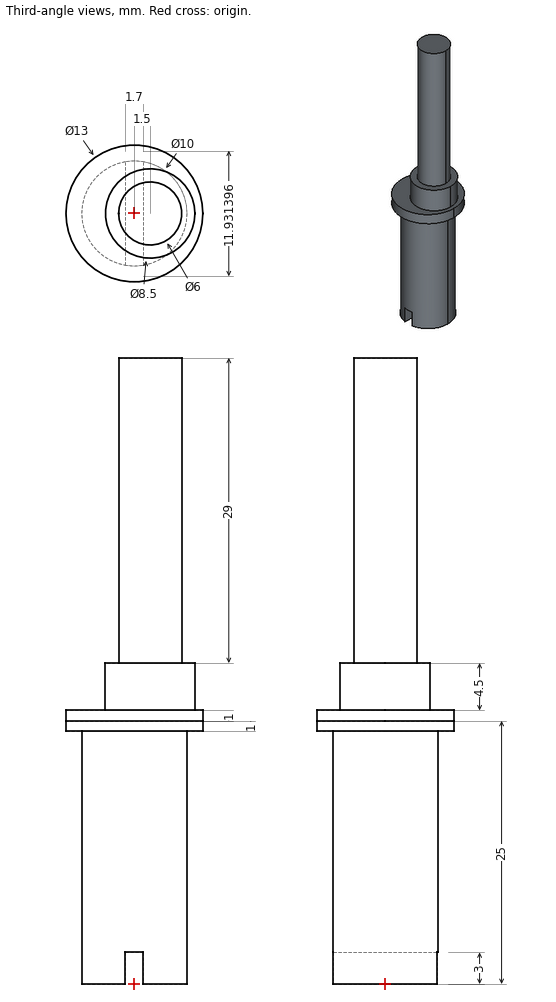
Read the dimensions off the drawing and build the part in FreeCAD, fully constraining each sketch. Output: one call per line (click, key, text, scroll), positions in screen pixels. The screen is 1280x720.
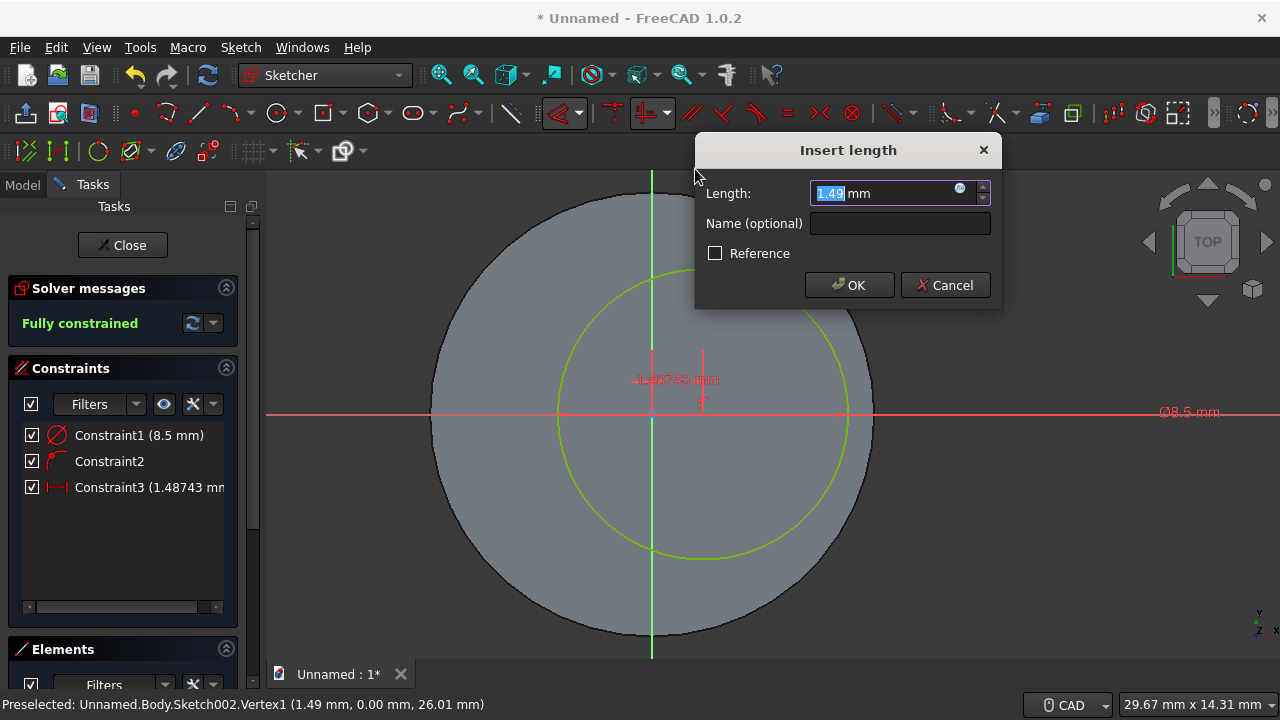
text(1.5)
key(Return)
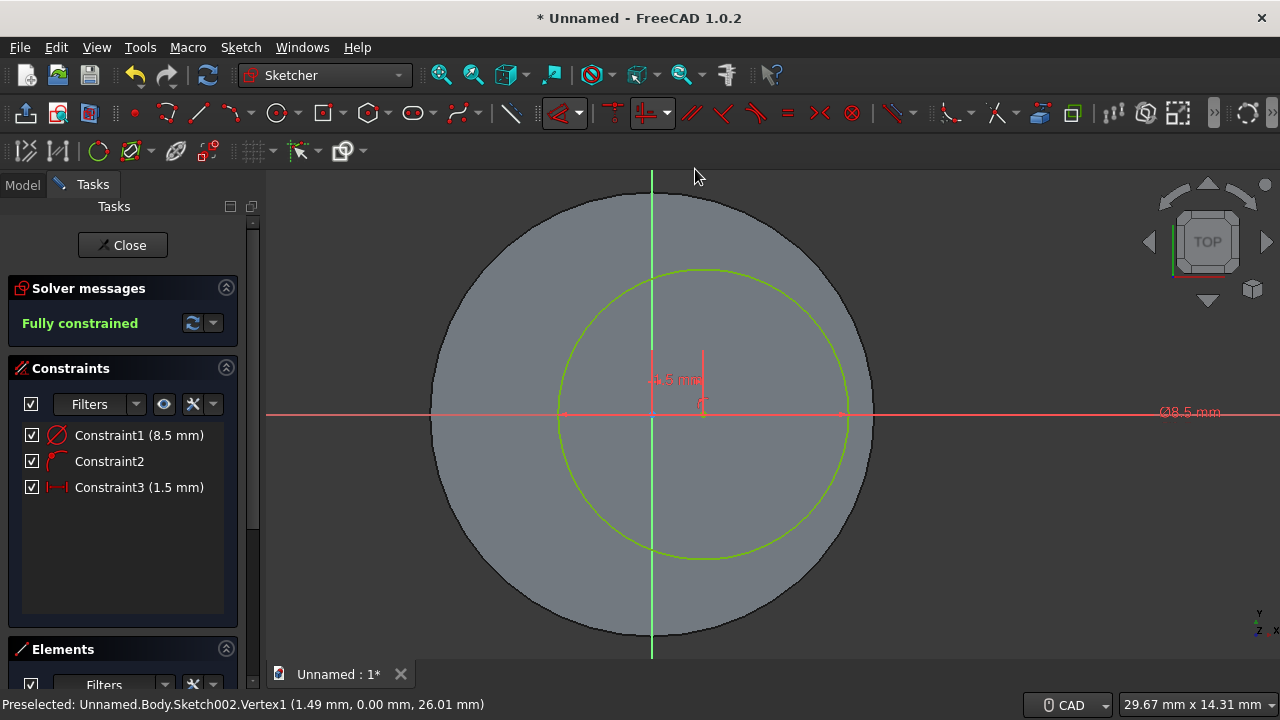
click(123, 245)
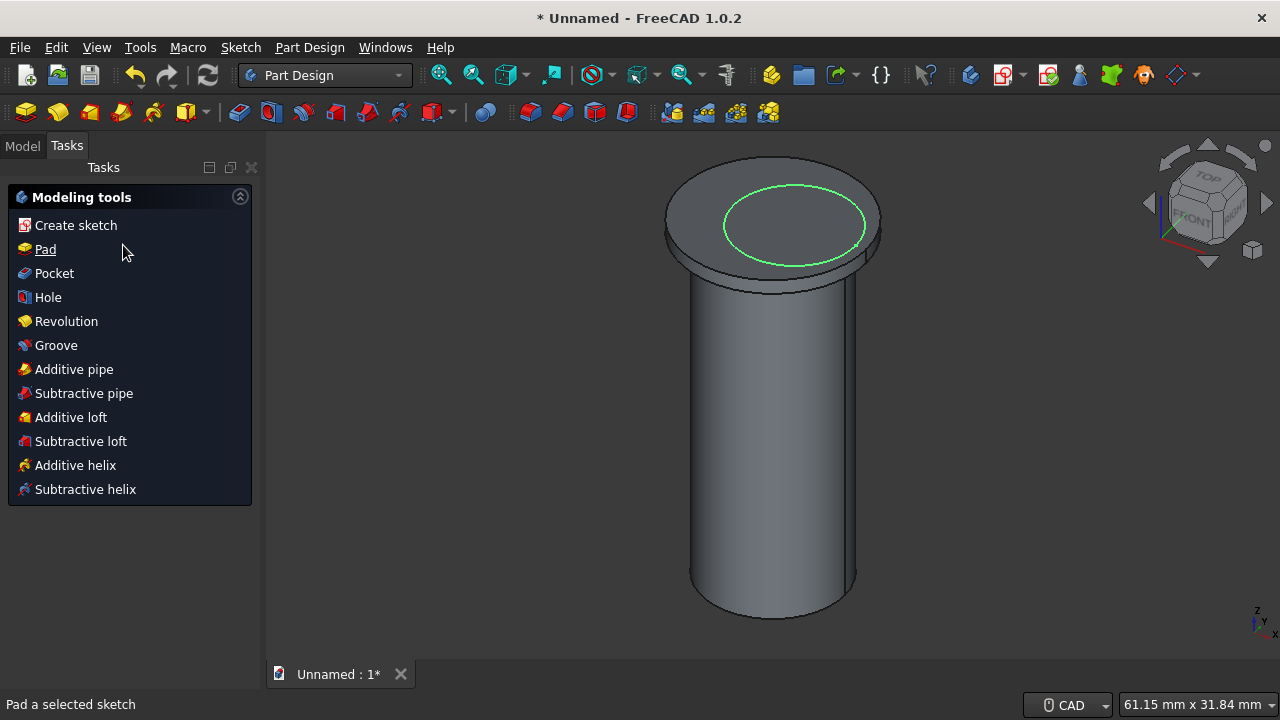
click(26, 112)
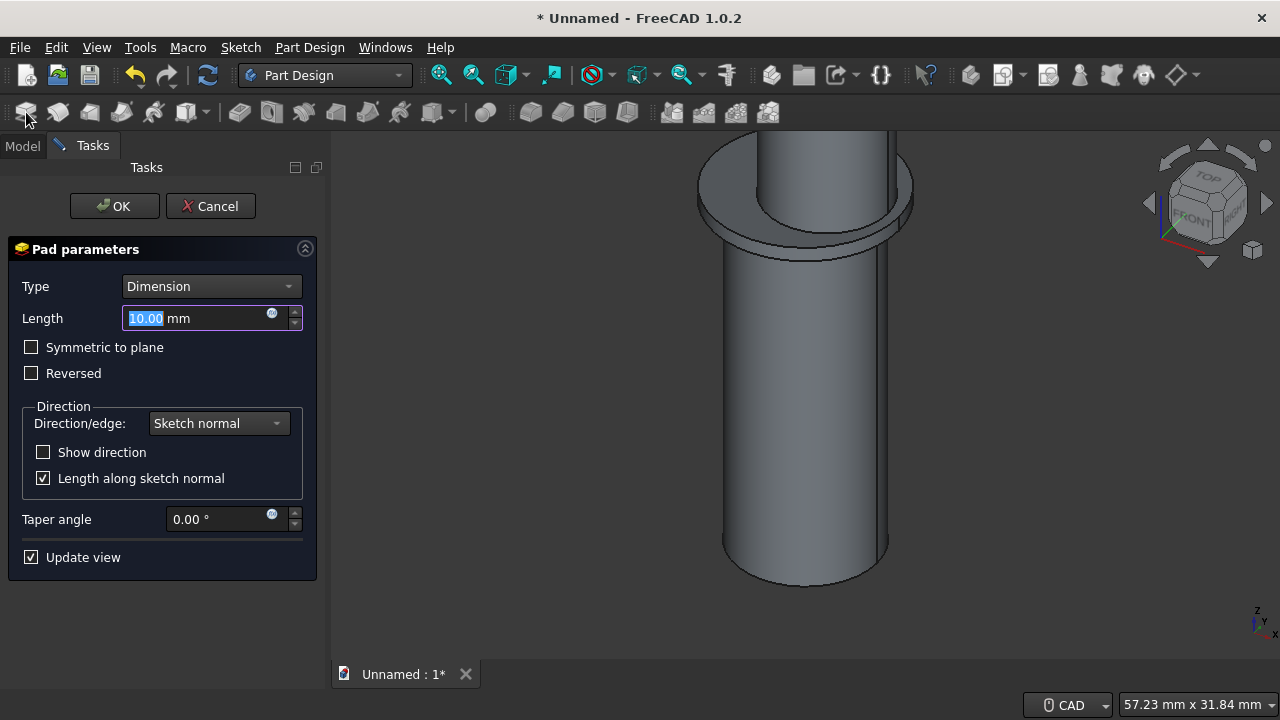
text(4.5)
key(Tab)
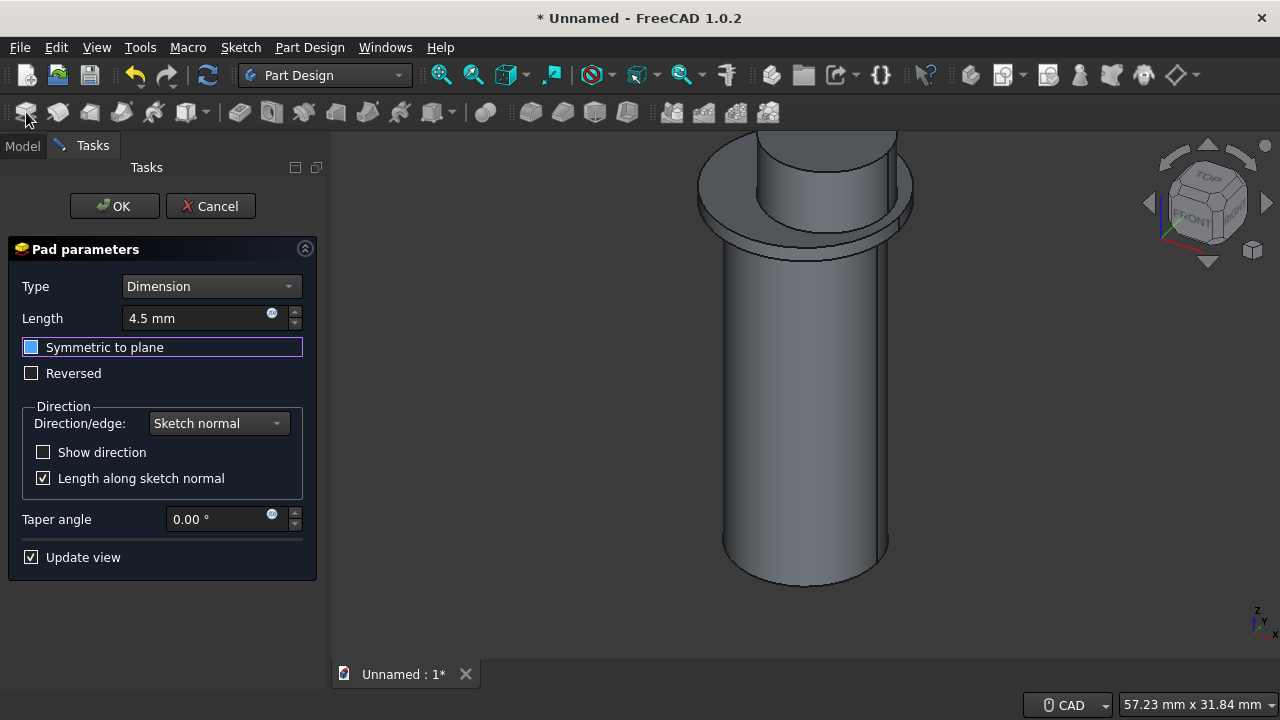
click(115, 206)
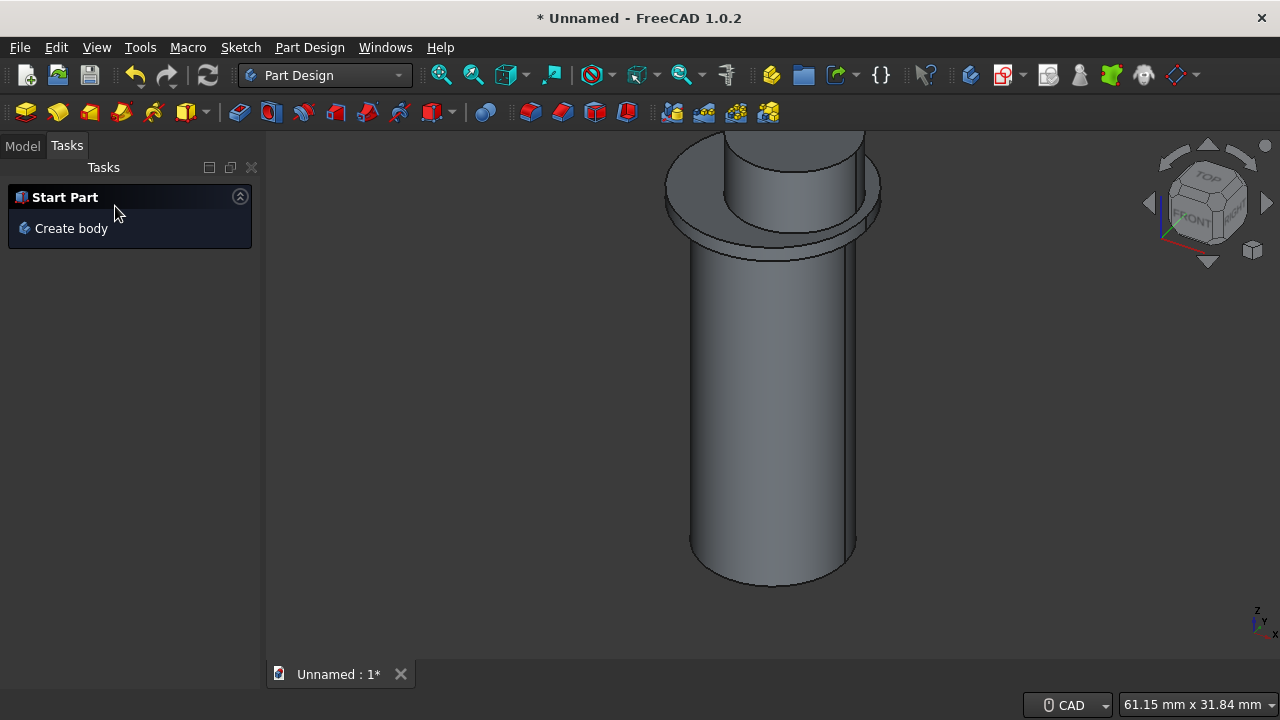
click(442, 76)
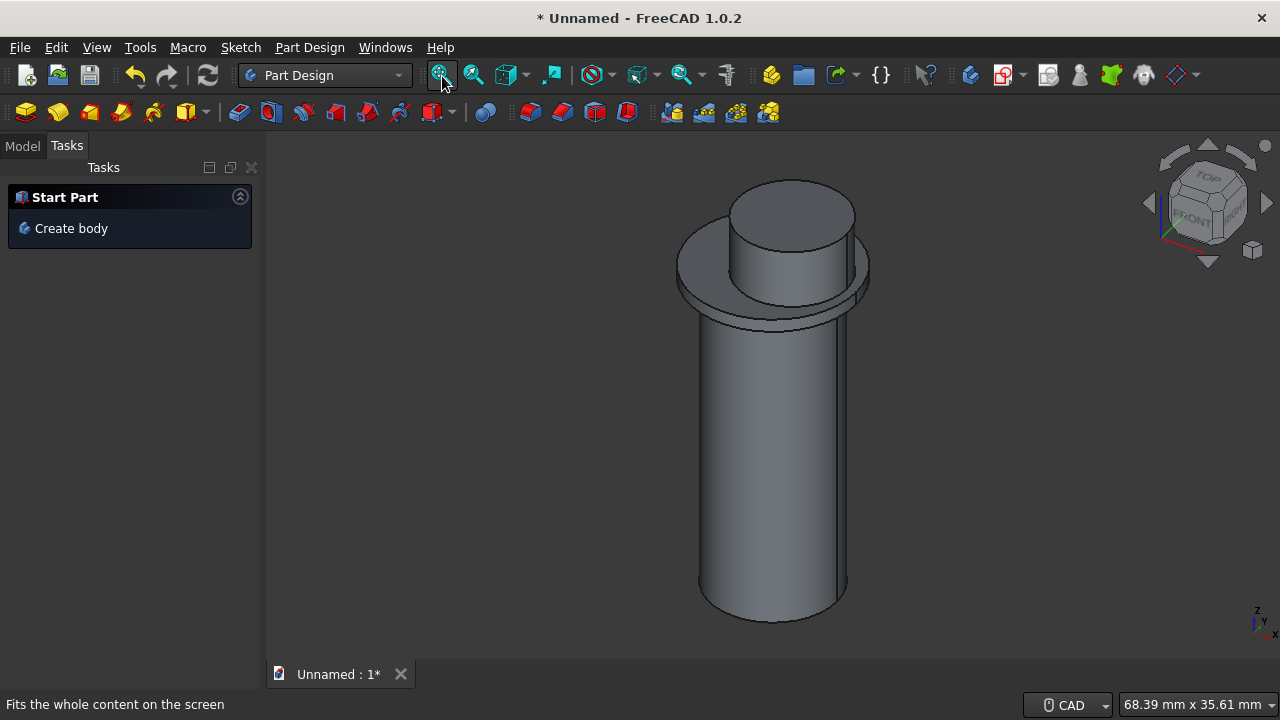
click(792, 215)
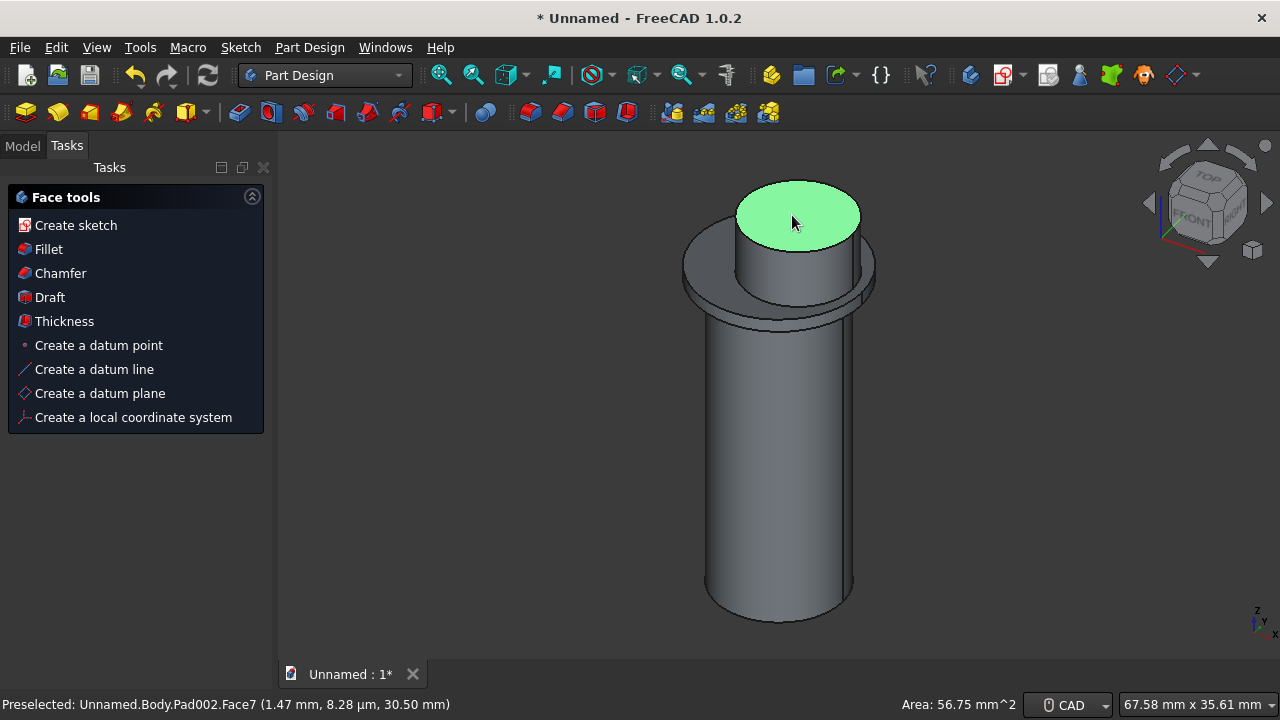
click(1004, 76)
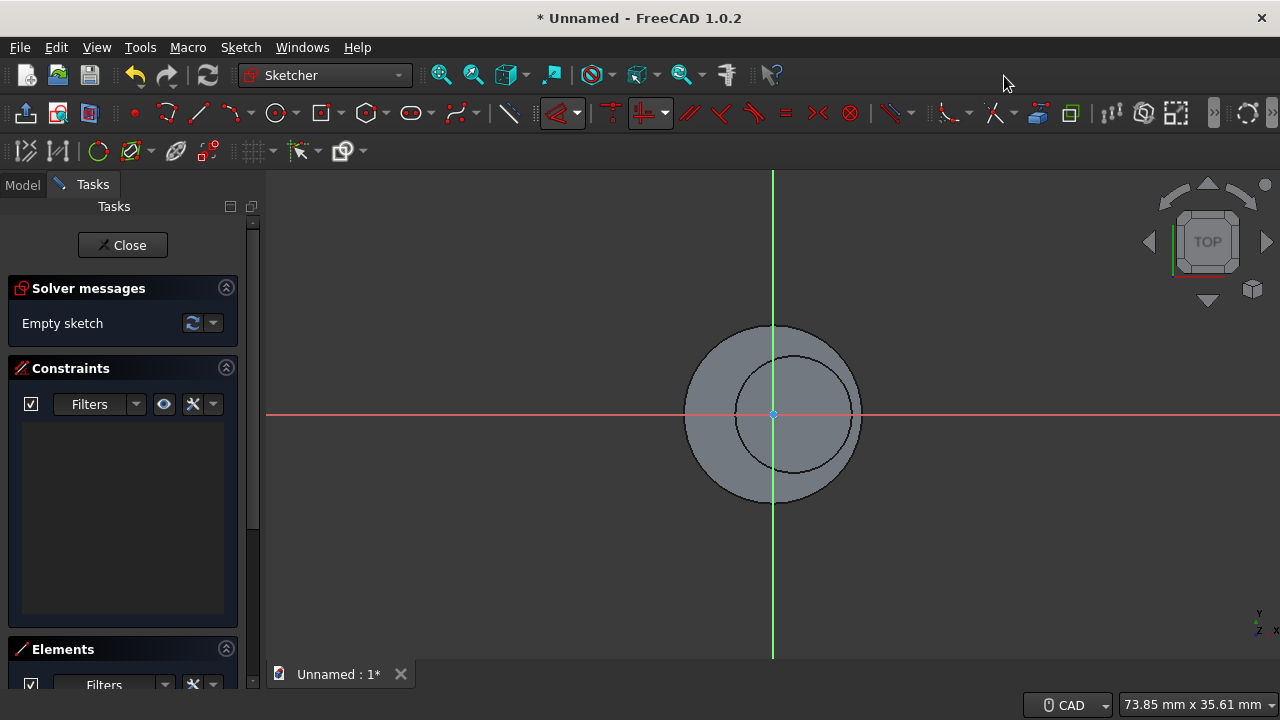
scroll(823, 415, up, 7)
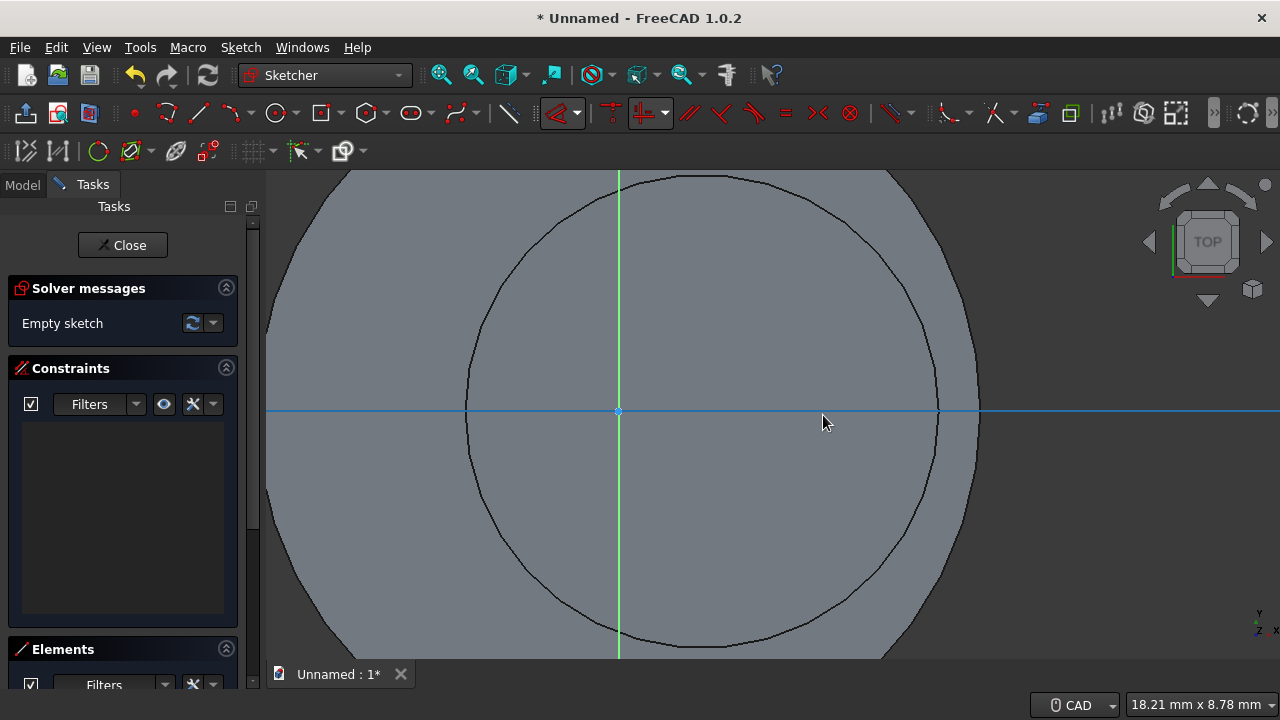
click(276, 114)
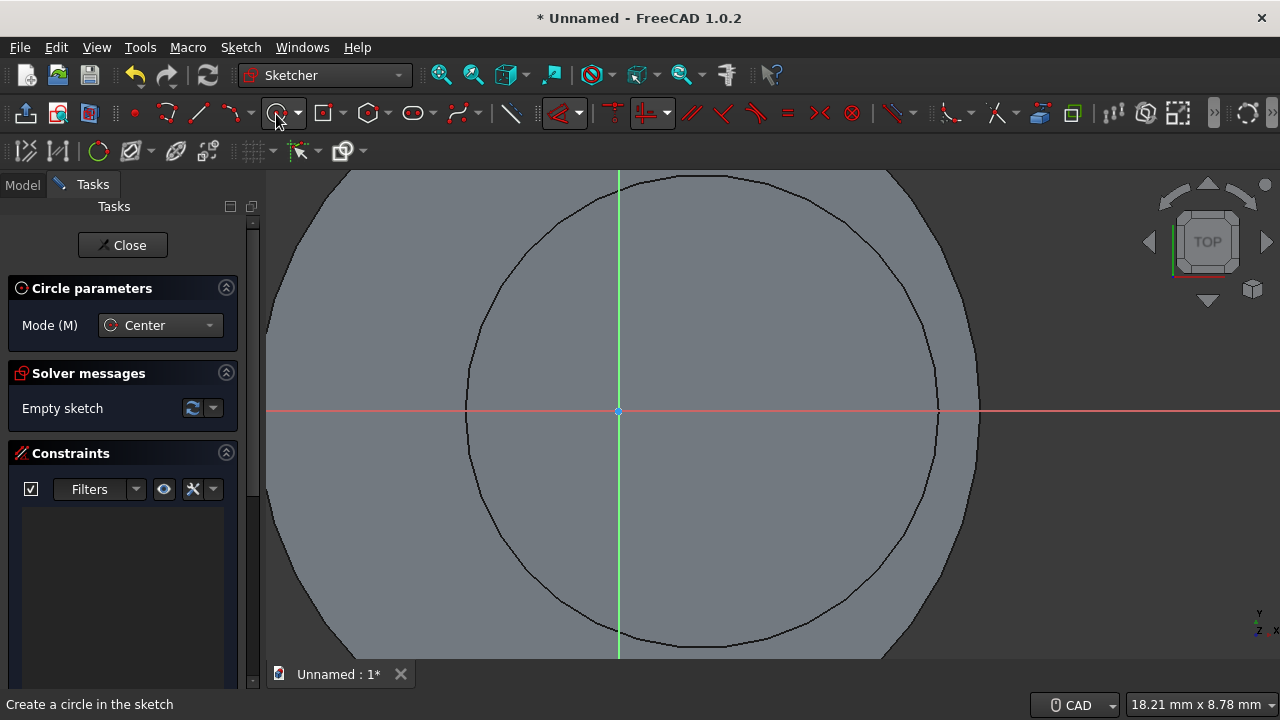
click(702, 411)
move(820, 293)